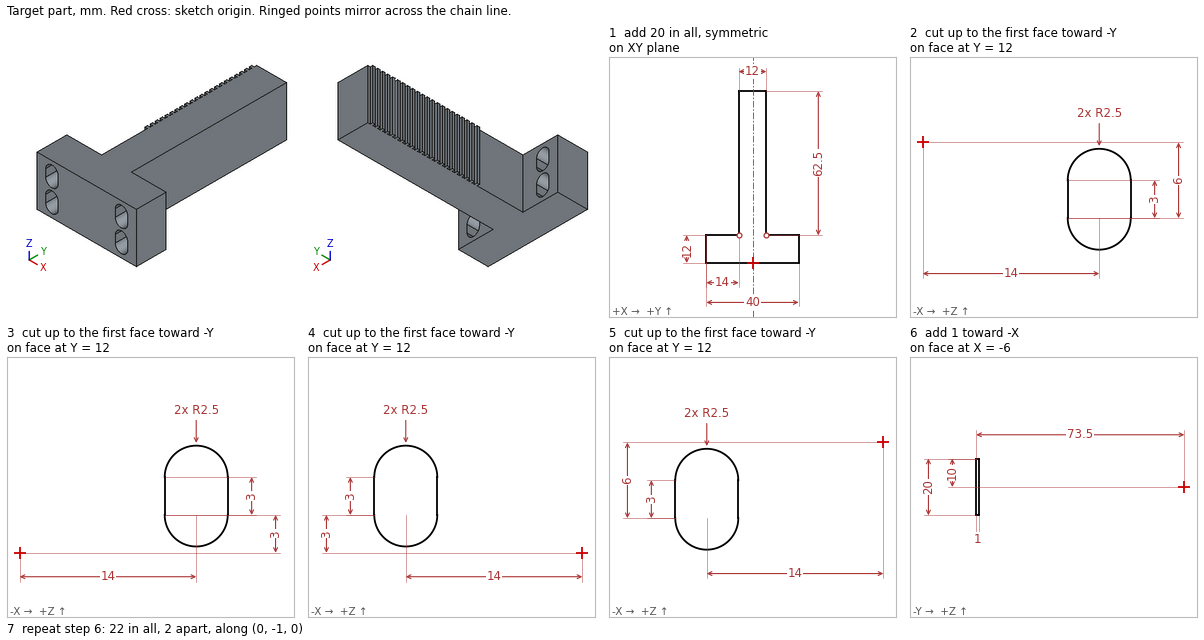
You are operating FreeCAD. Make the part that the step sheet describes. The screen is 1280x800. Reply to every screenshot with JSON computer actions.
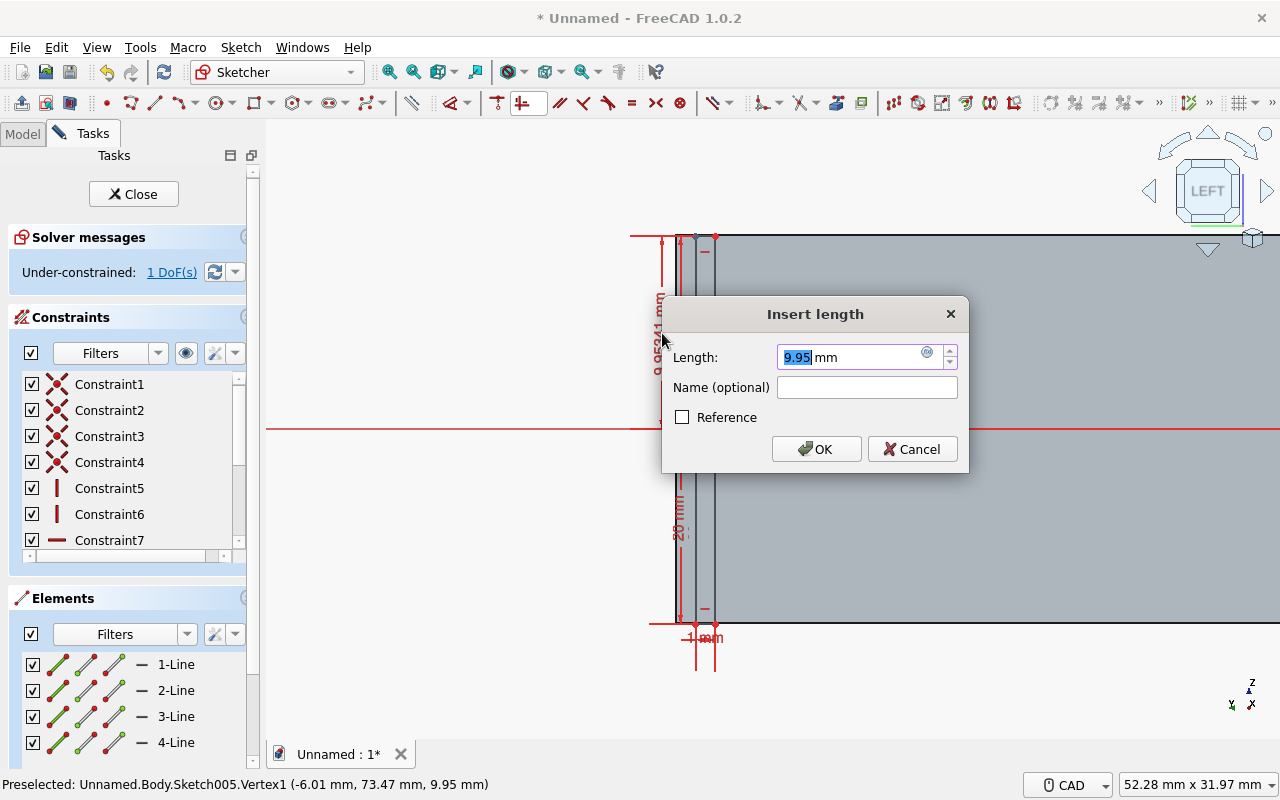
{"action": "type", "text": "10"}
{"action": "key", "text": "Return"}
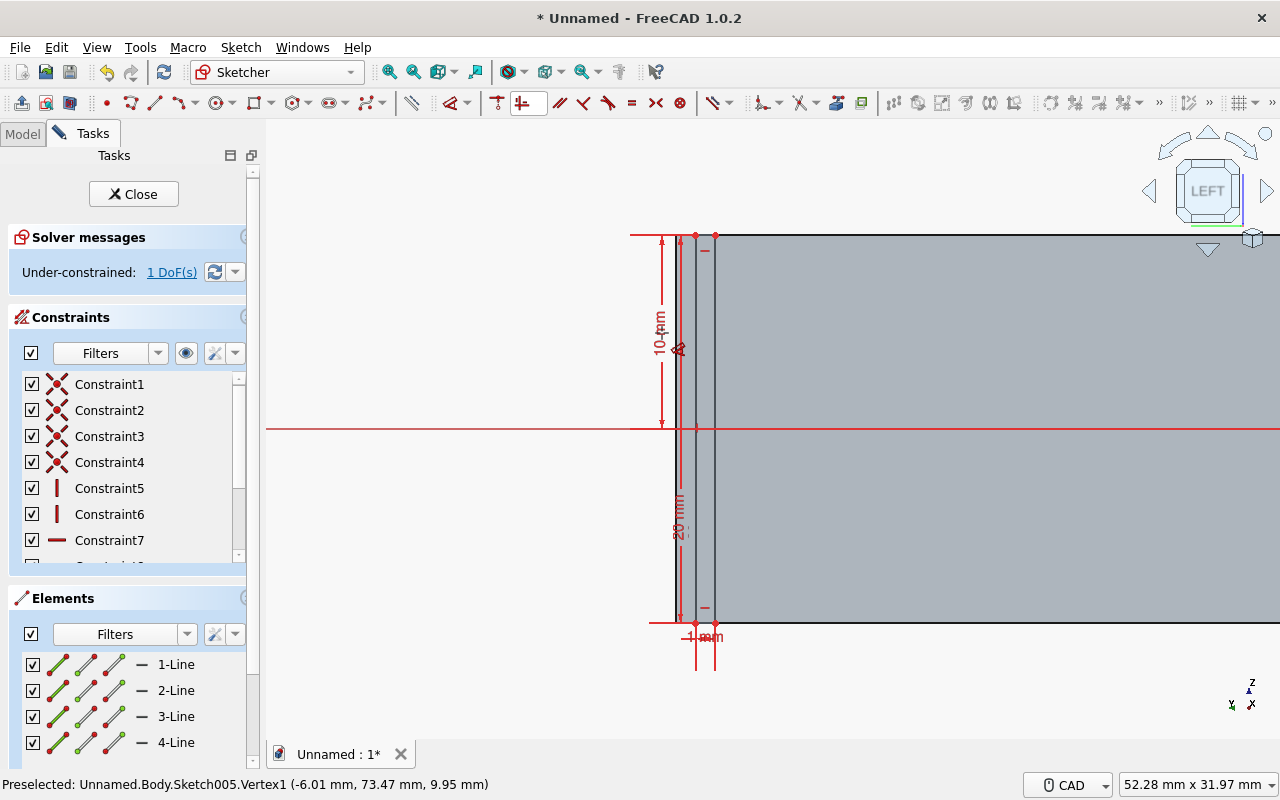
{"action": "left_click", "coordinate": [696, 235]}
{"action": "left_click", "coordinate": [905, 201]}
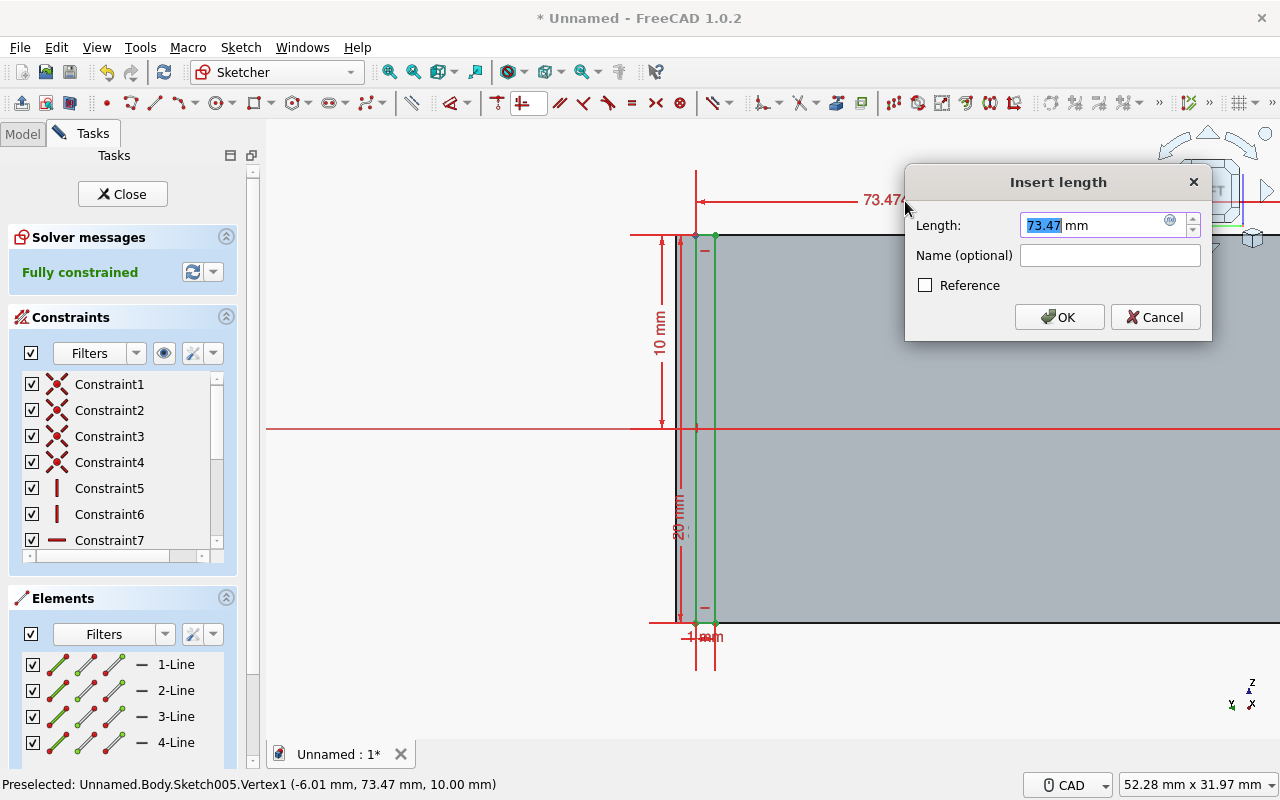
{"action": "type", "text": "73.5"}
{"action": "key", "text": "Return"}
{"action": "key", "text": "Escape"}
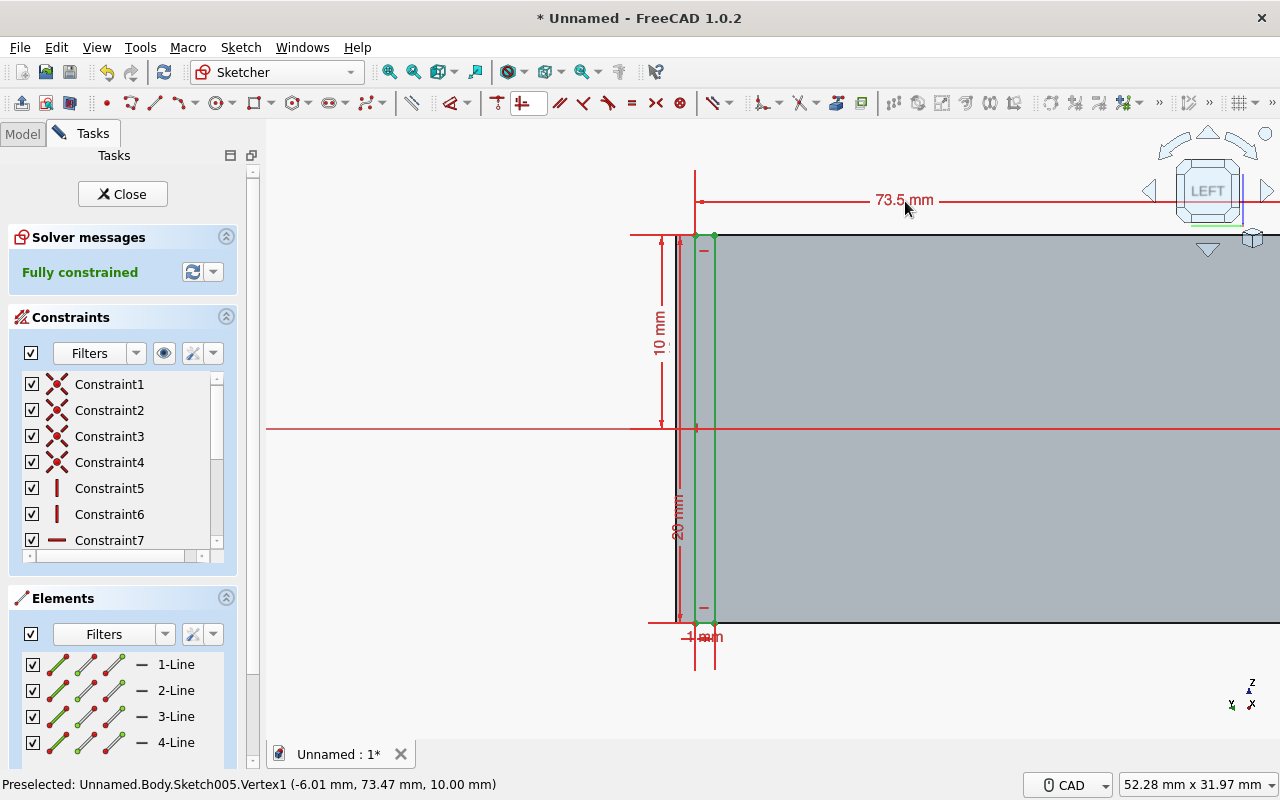
{"action": "left_click", "coordinate": [123, 194]}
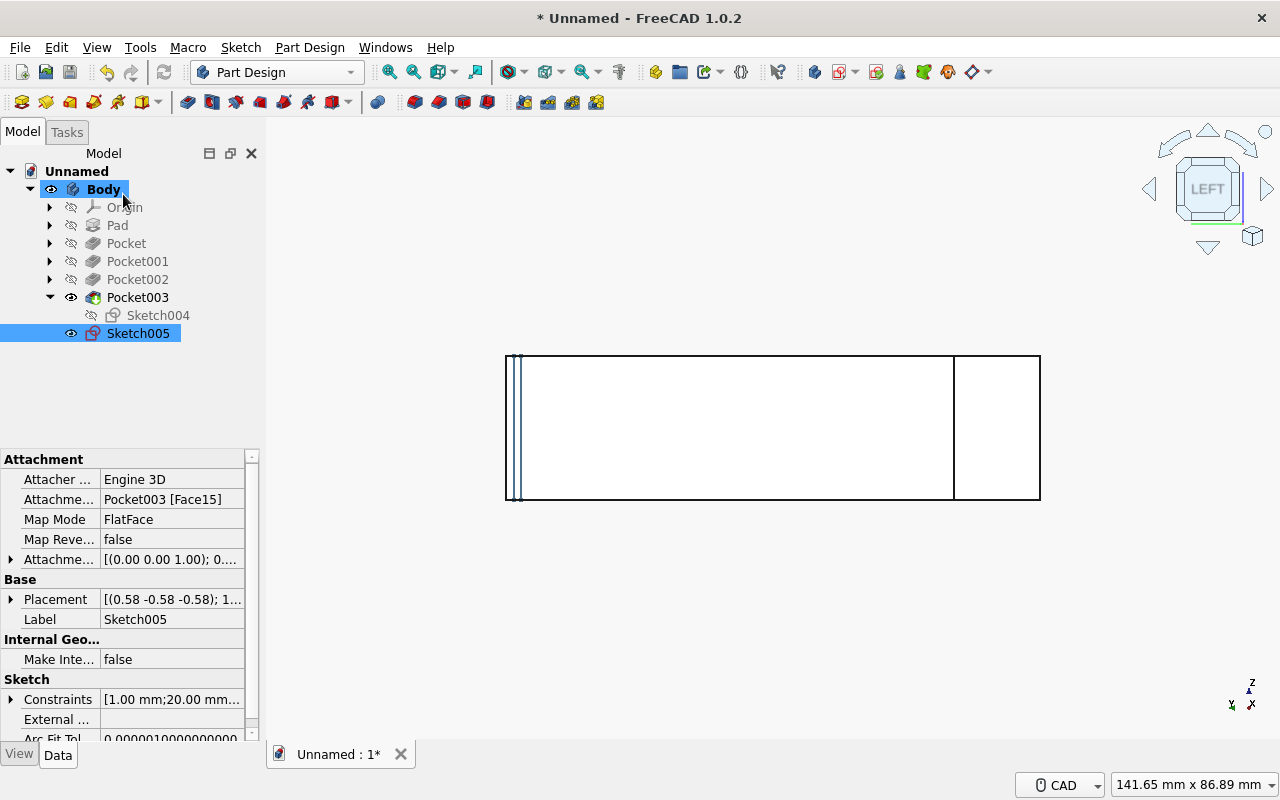
{"action": "left_click", "coordinate": [22, 102]}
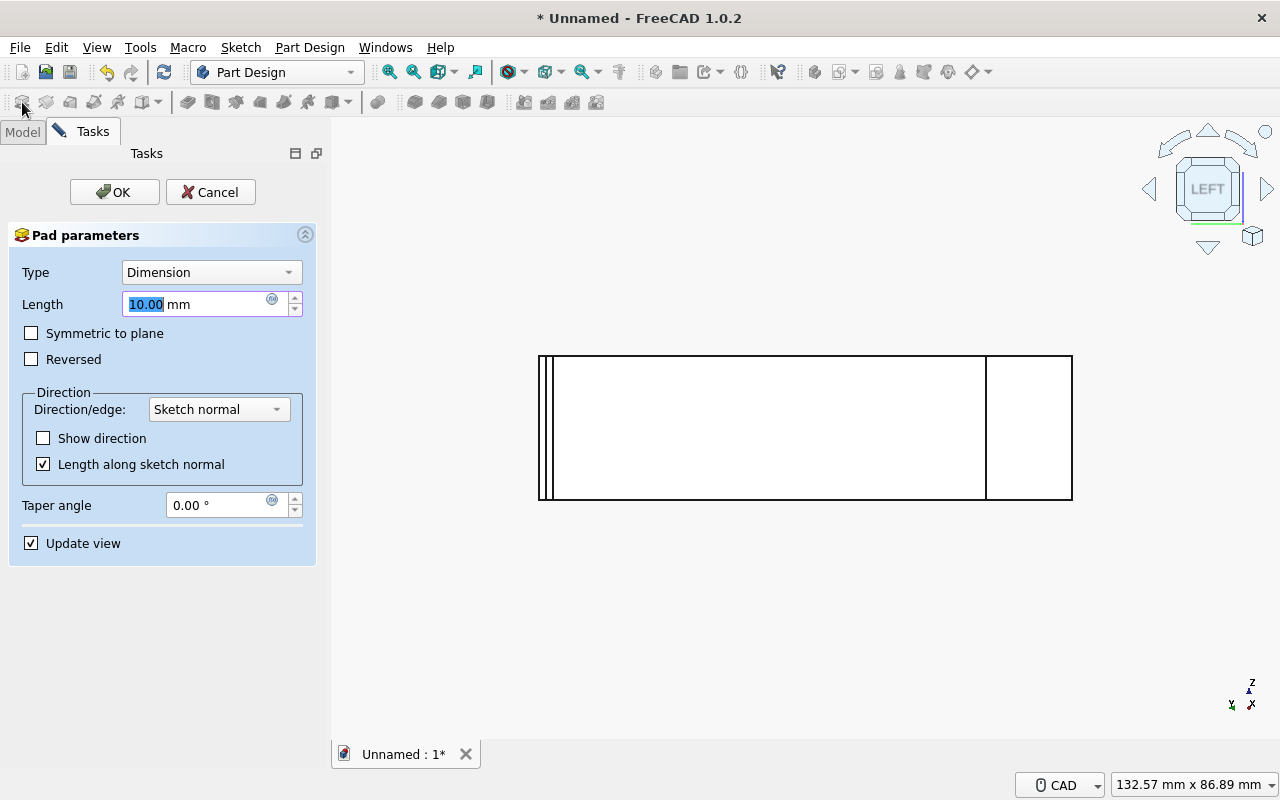
{"action": "type", "text": "1"}
{"action": "key", "text": "Tab"}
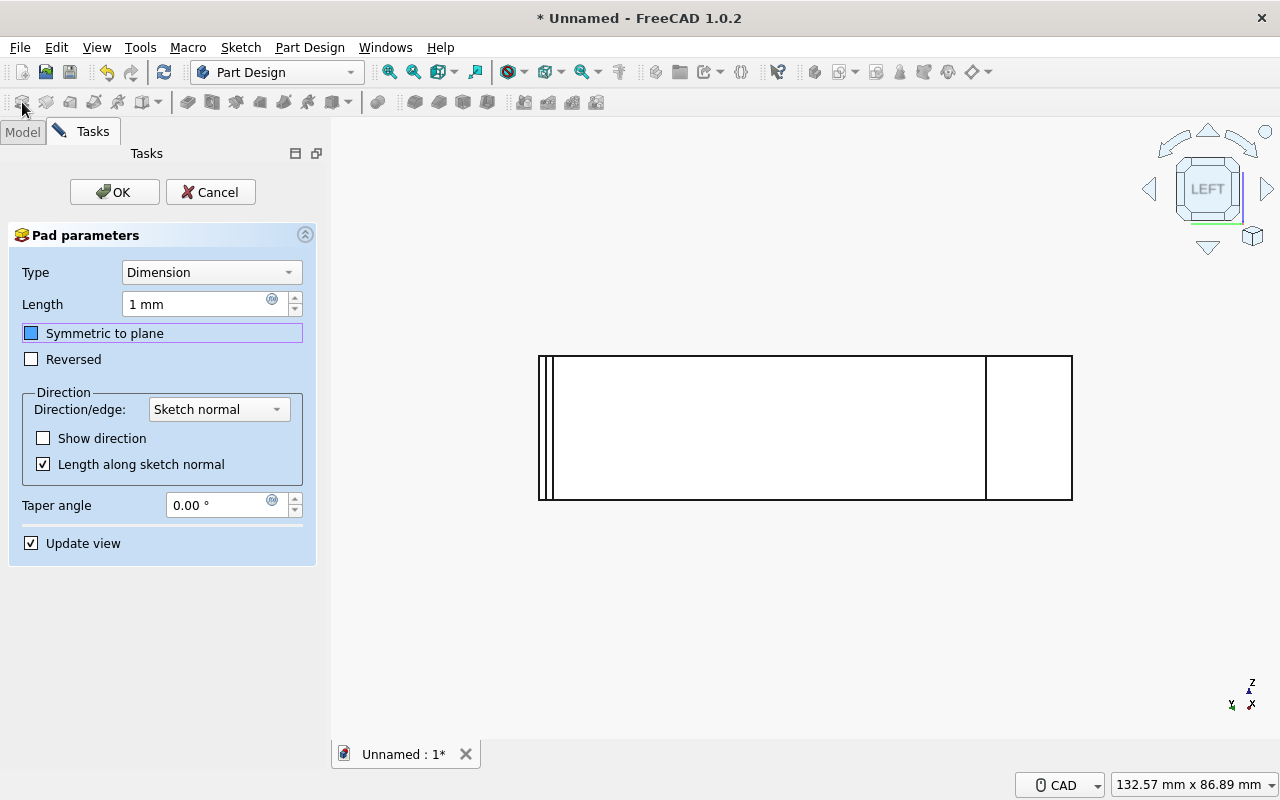
{"action": "left_click", "coordinate": [115, 192]}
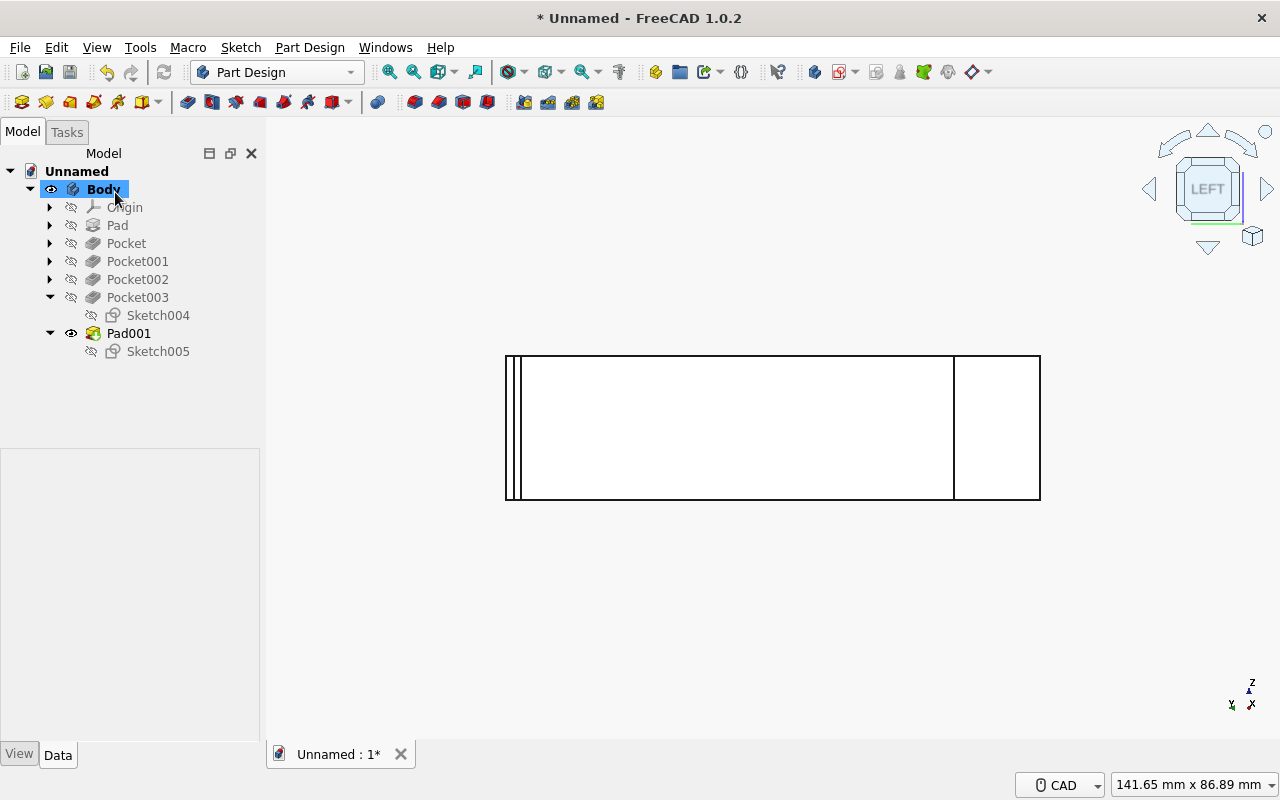
{"action": "left_click", "coordinate": [116, 333]}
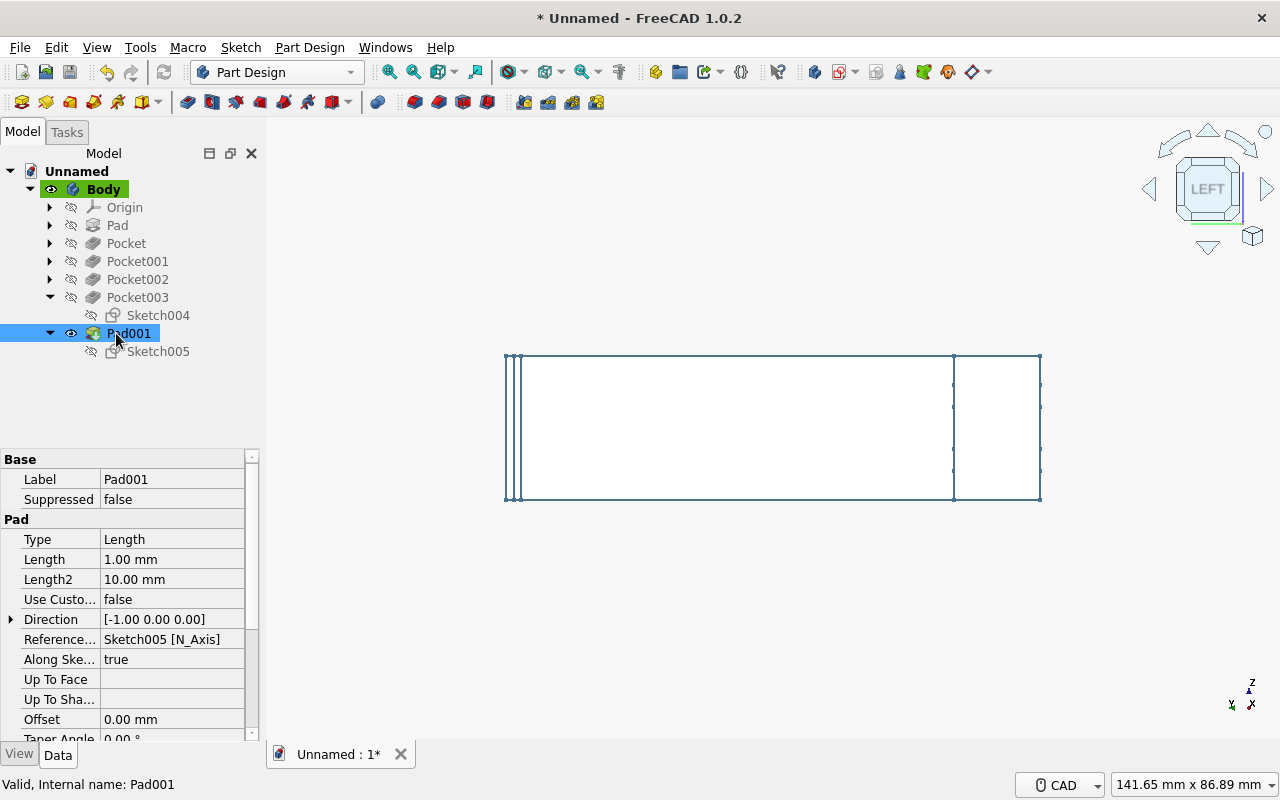
{"action": "left_click", "coordinate": [548, 102]}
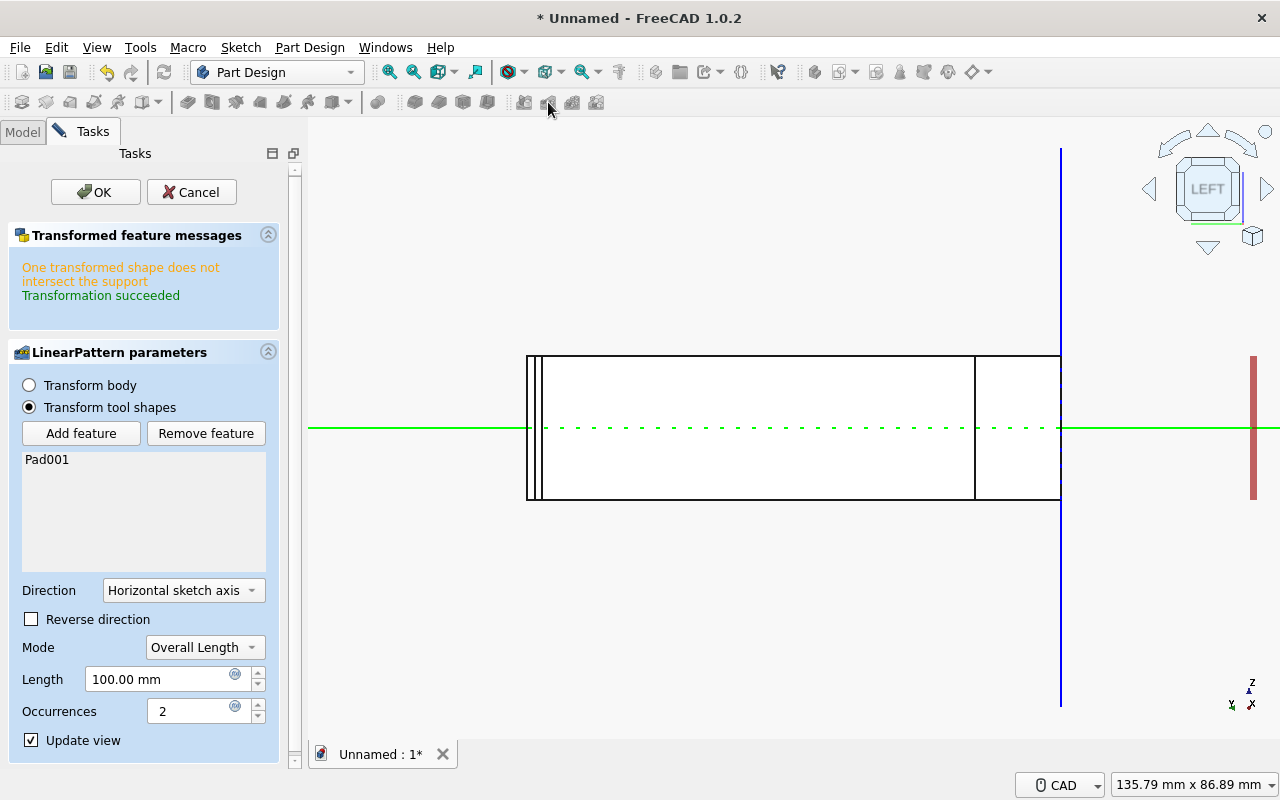
{"action": "left_click", "coordinate": [184, 590]}